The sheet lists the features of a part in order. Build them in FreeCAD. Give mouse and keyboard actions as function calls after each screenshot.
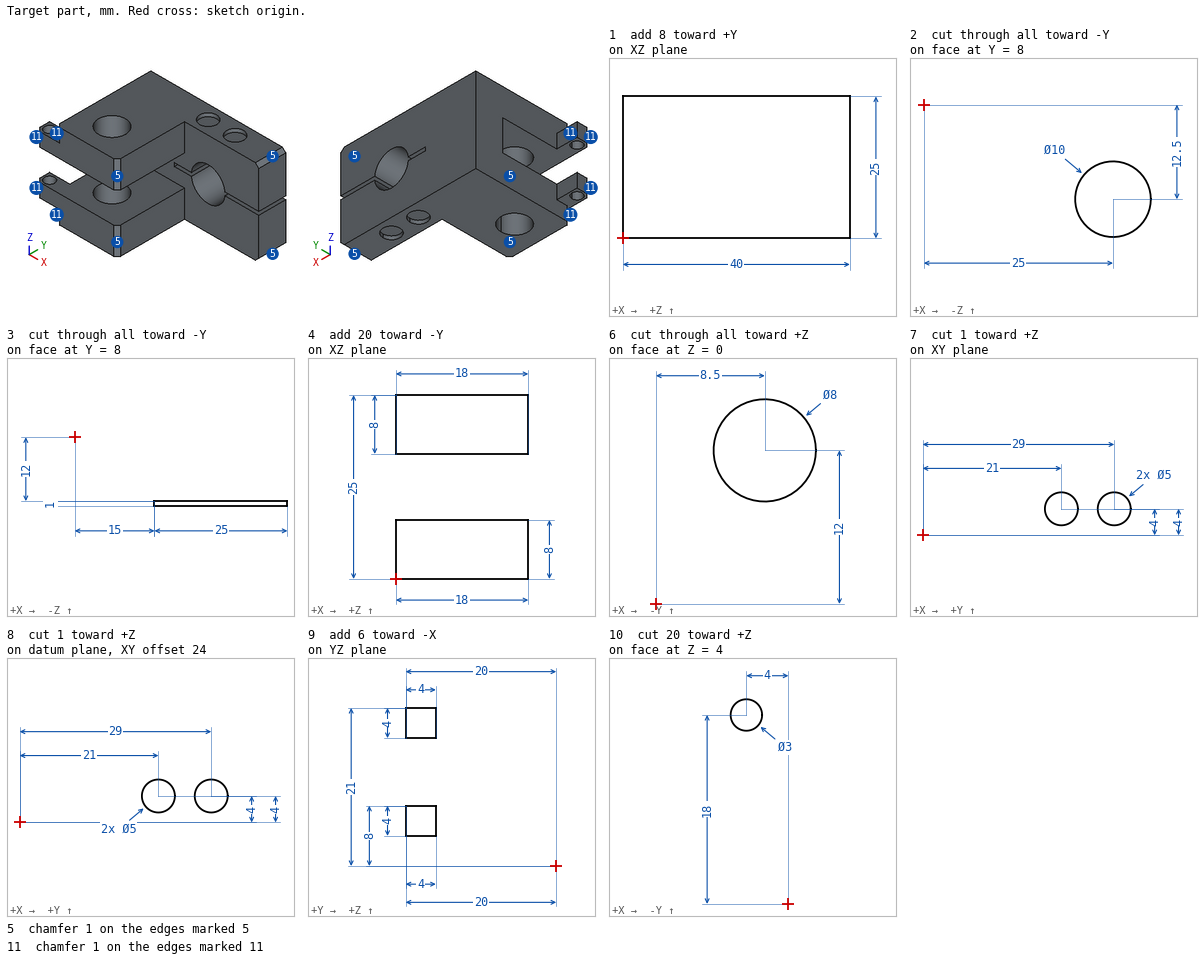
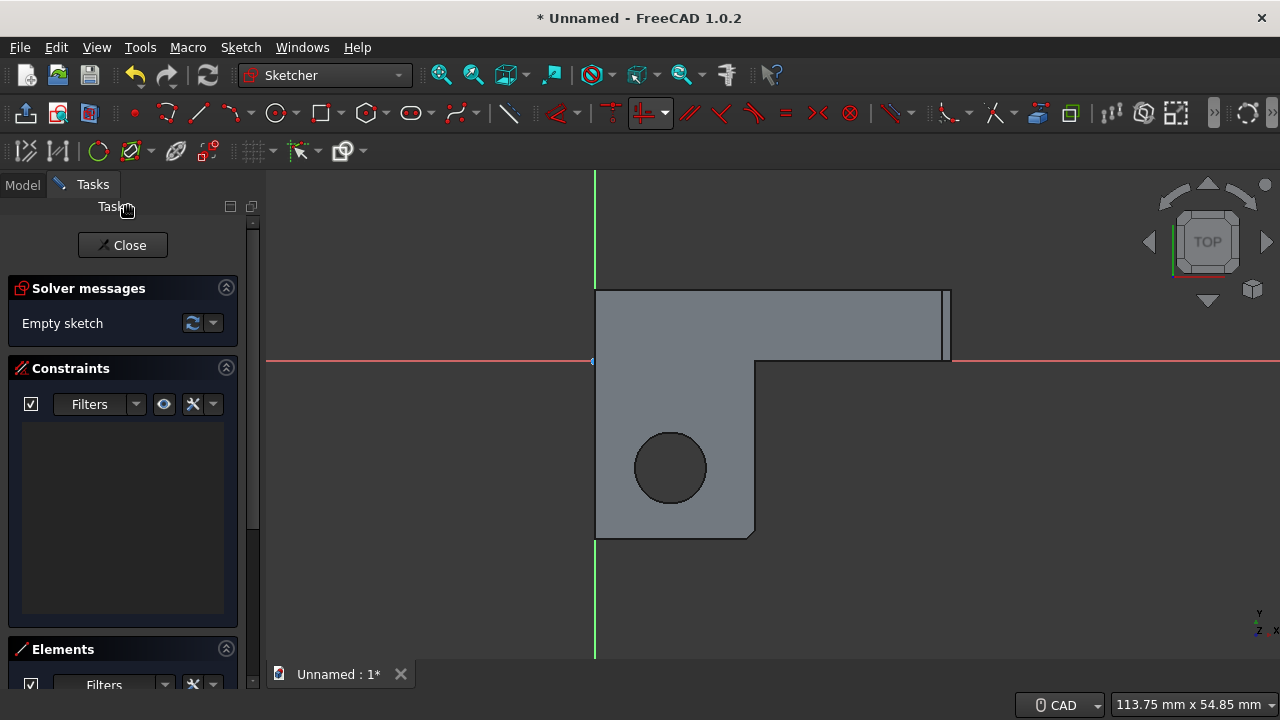
click(90, 114)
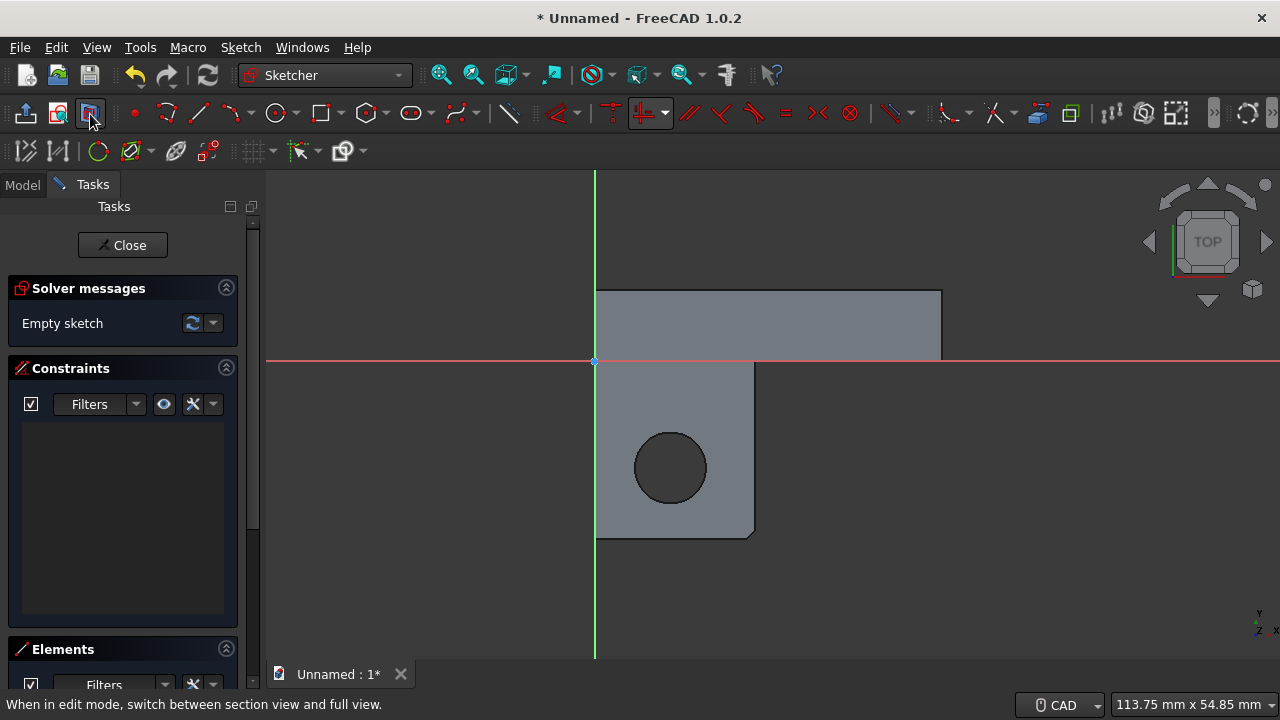
scroll(760, 265, up, 4)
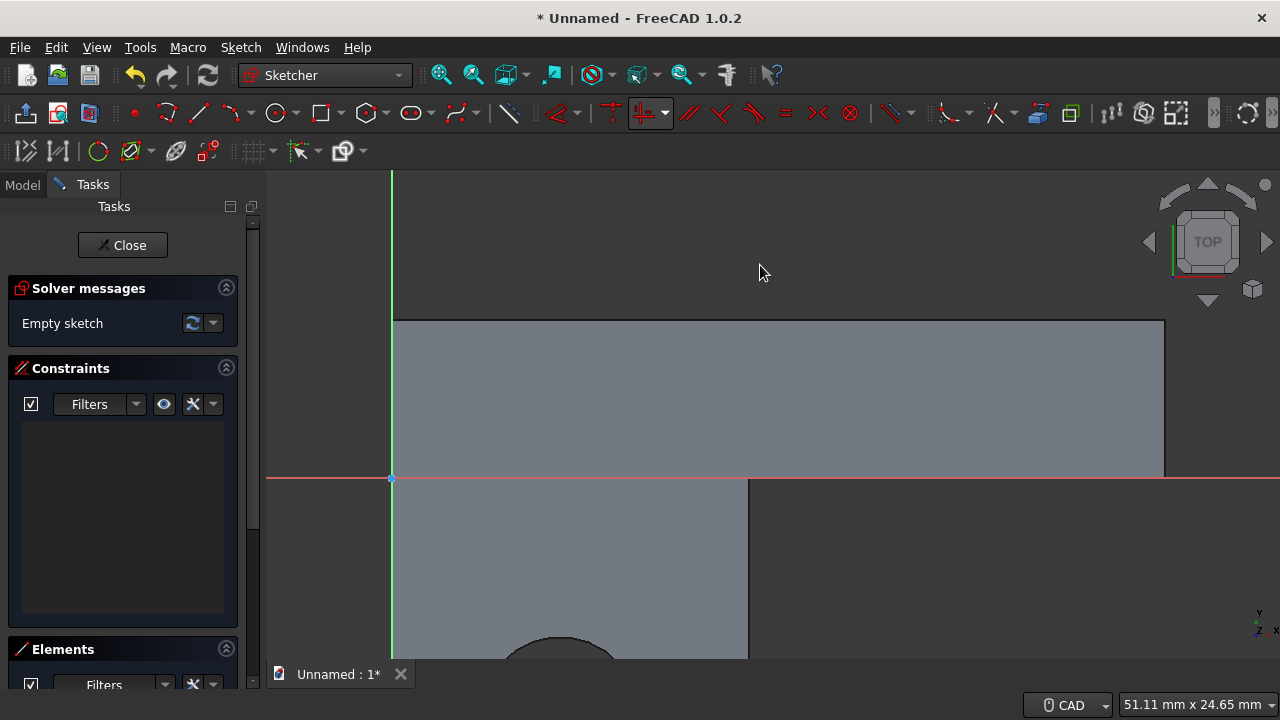
click(276, 114)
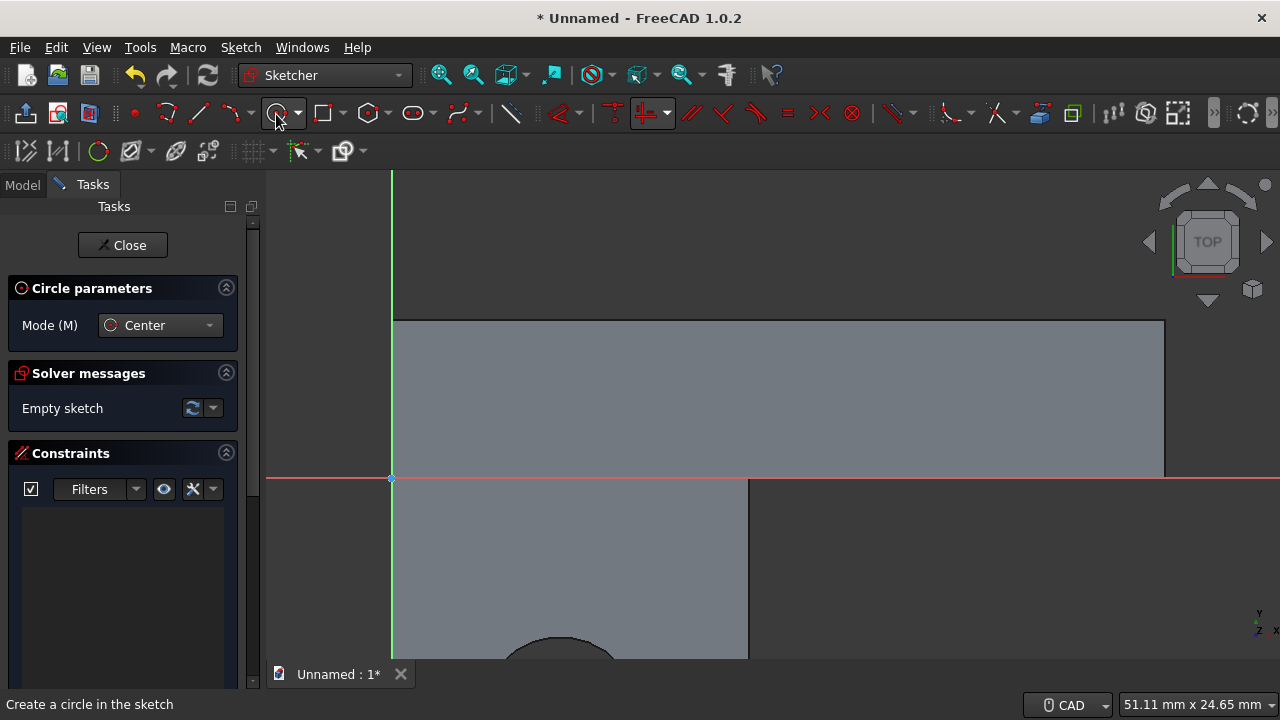
click(967, 399)
click(1002, 364)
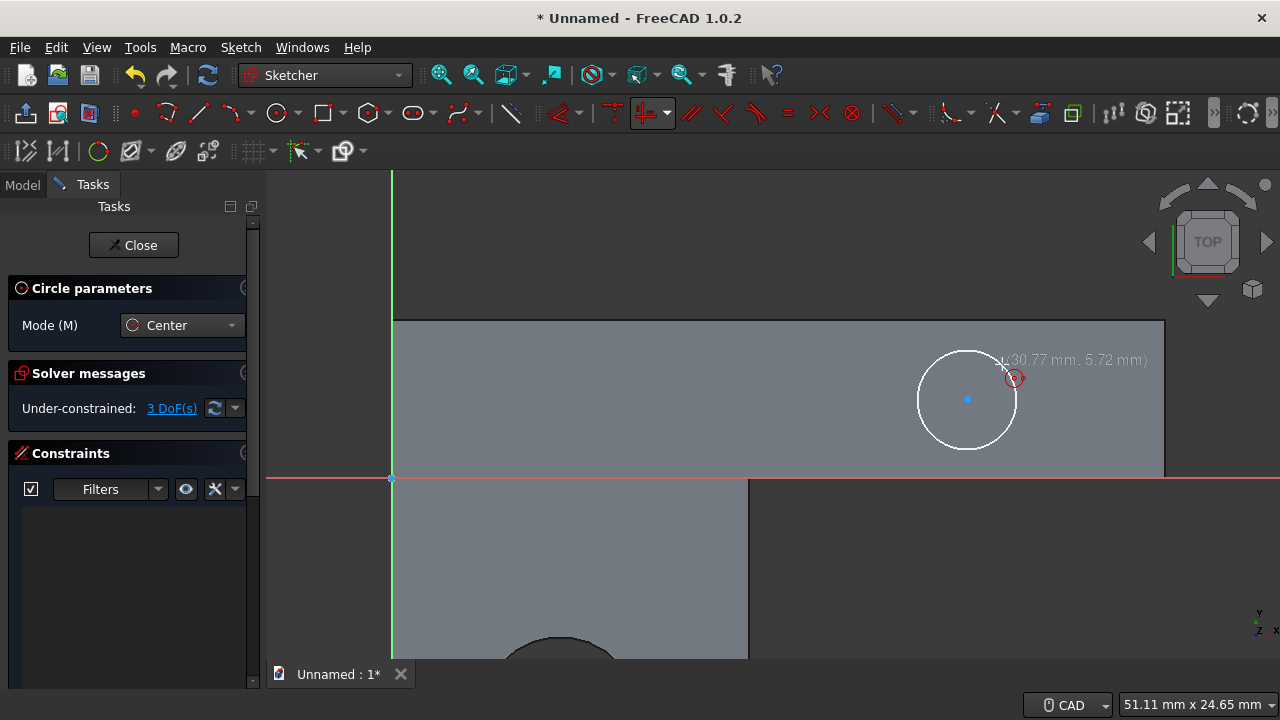
click(808, 399)
click(843, 364)
key(Escape)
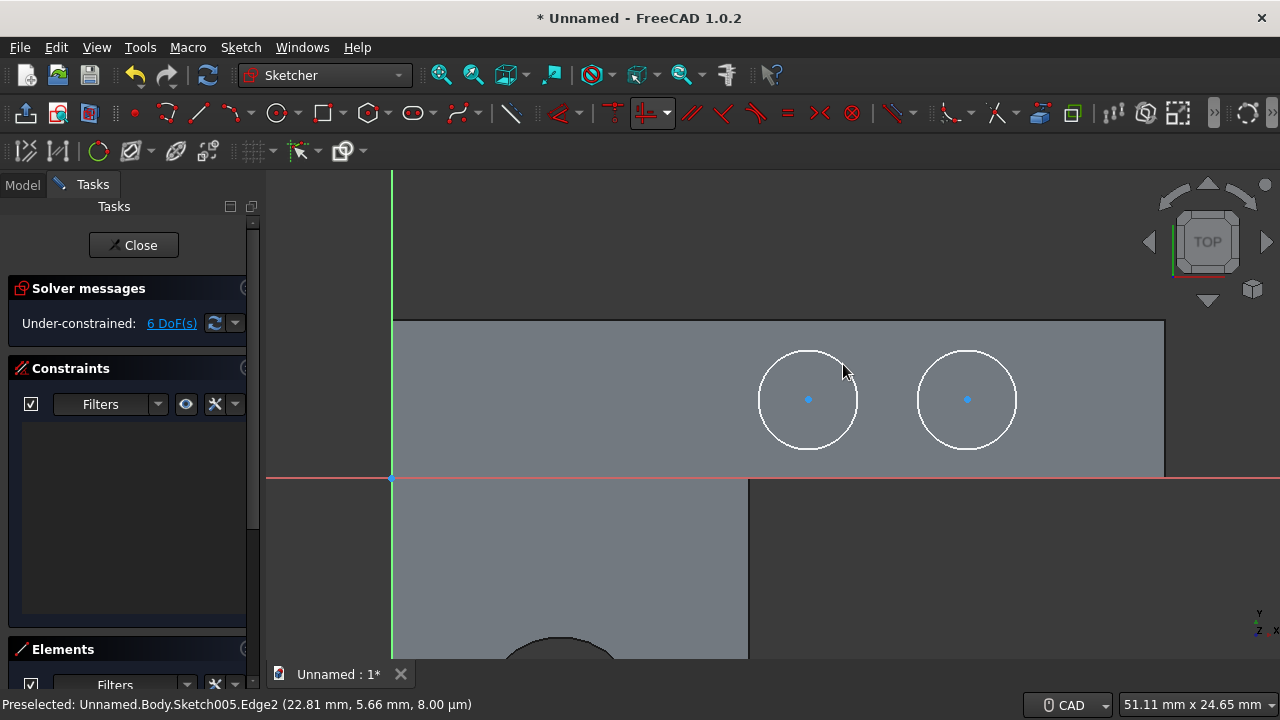
click(1002, 365)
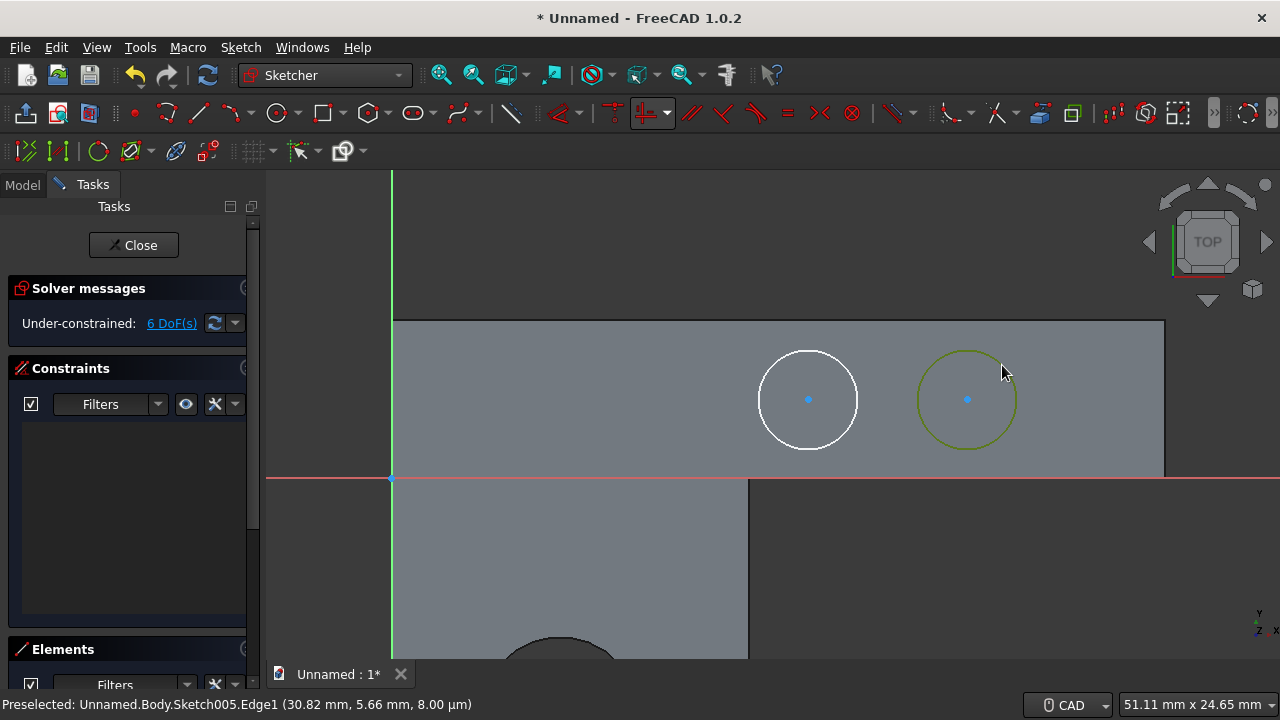
click(843, 365)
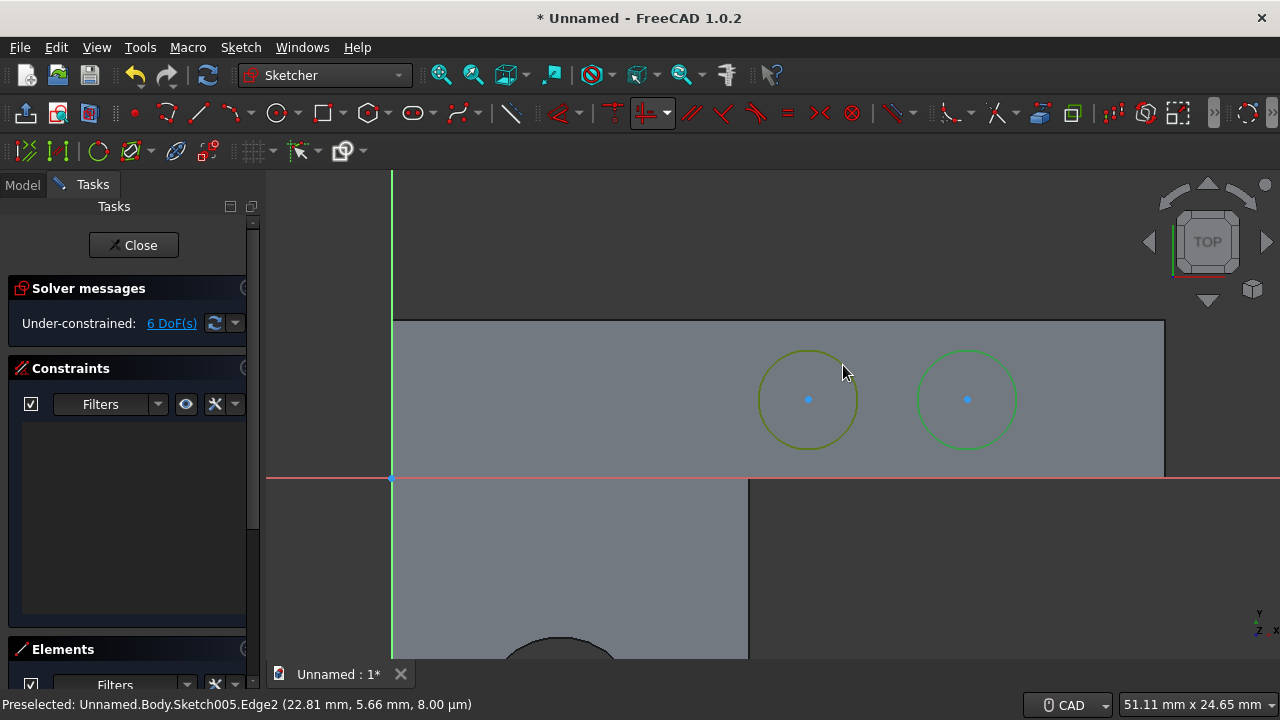
click(788, 114)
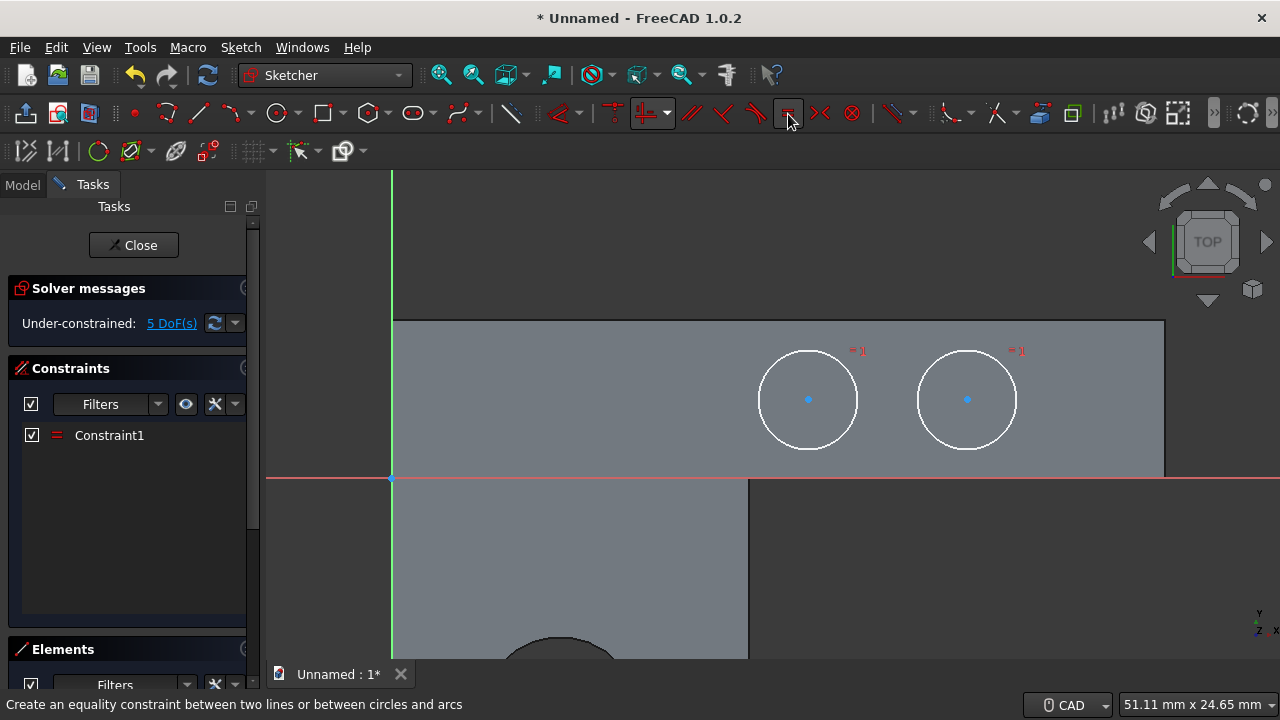
click(558, 114)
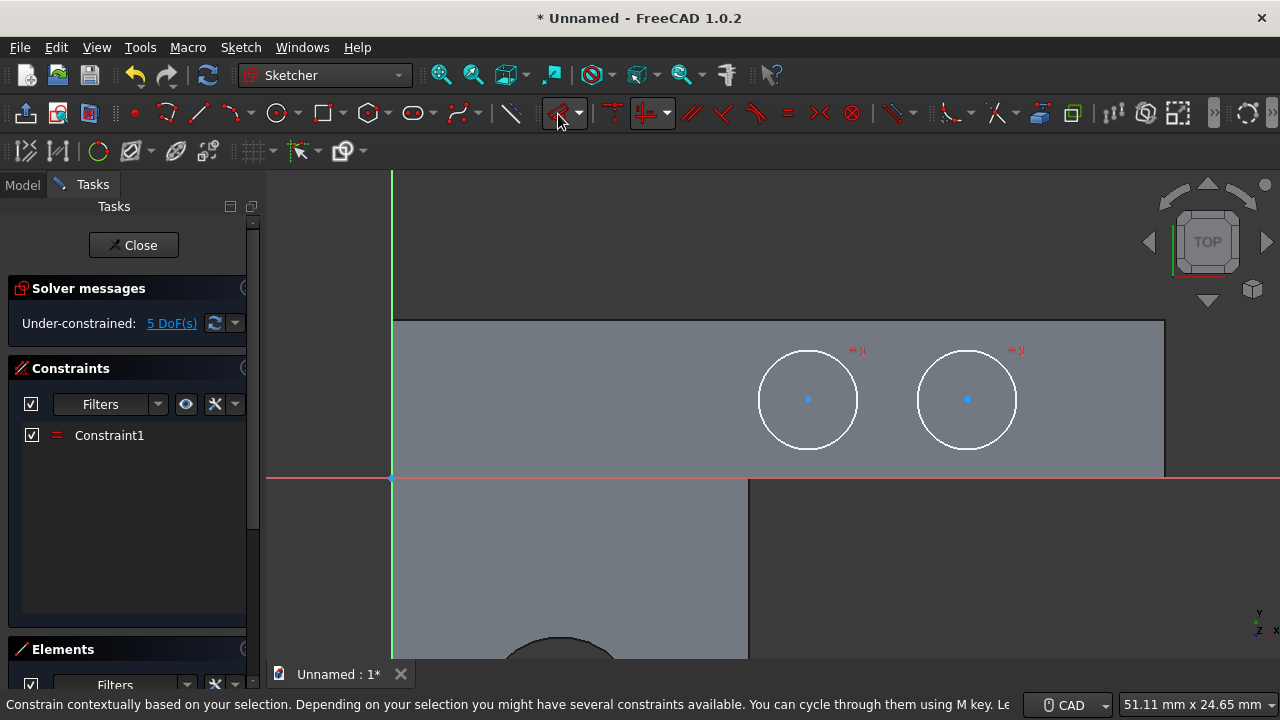
click(1002, 365)
click(1025, 342)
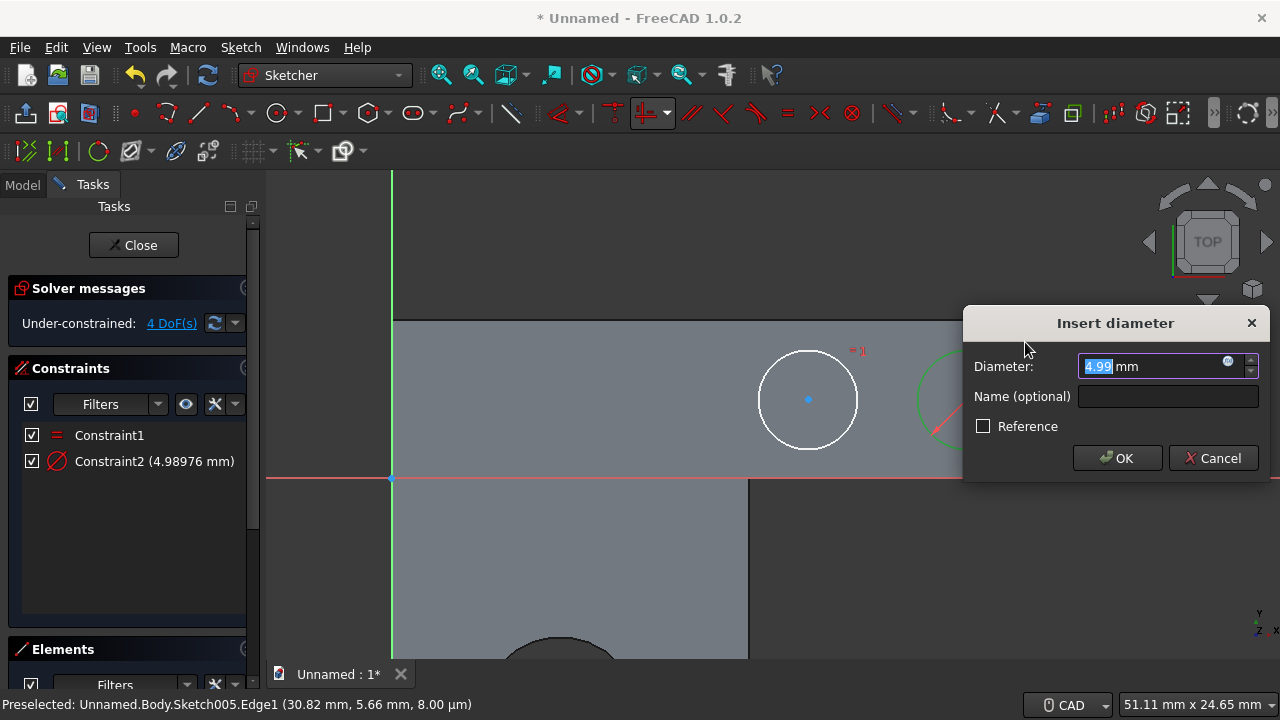
text(5)
key(Return)